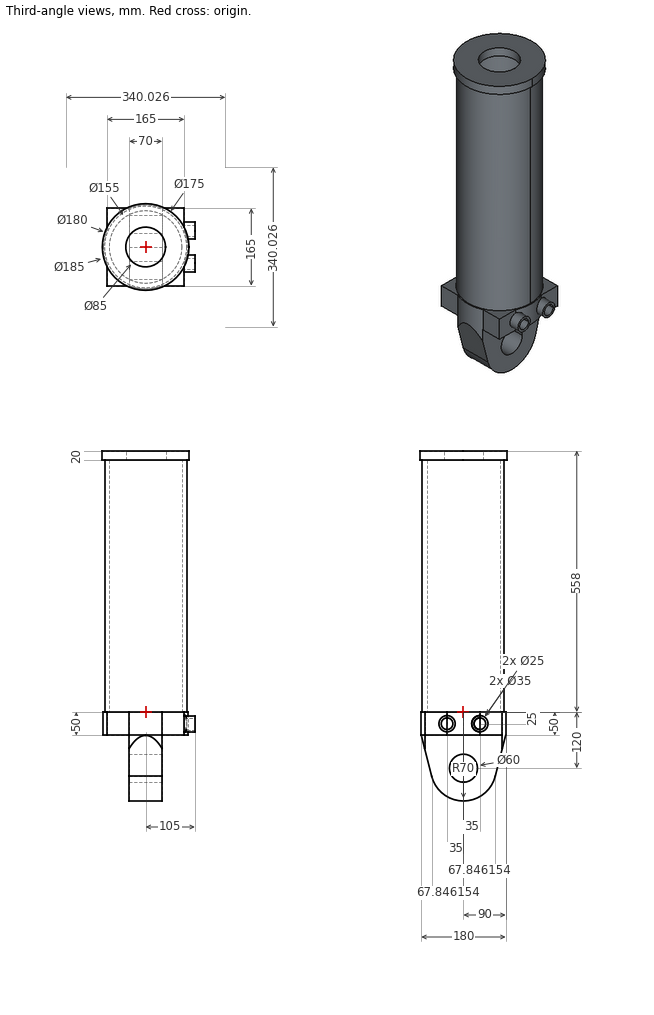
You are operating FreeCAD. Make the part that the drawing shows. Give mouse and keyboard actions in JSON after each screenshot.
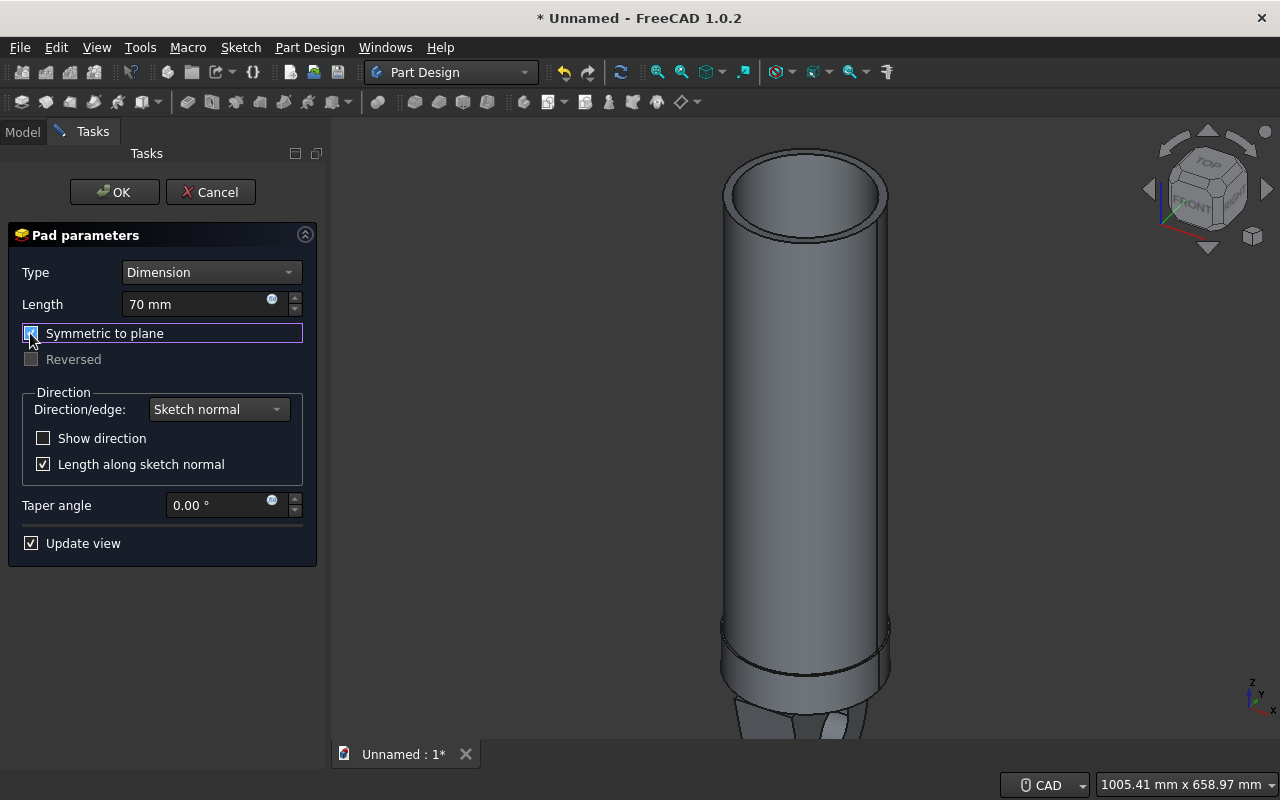
{"action": "left_click", "coordinate": [115, 192]}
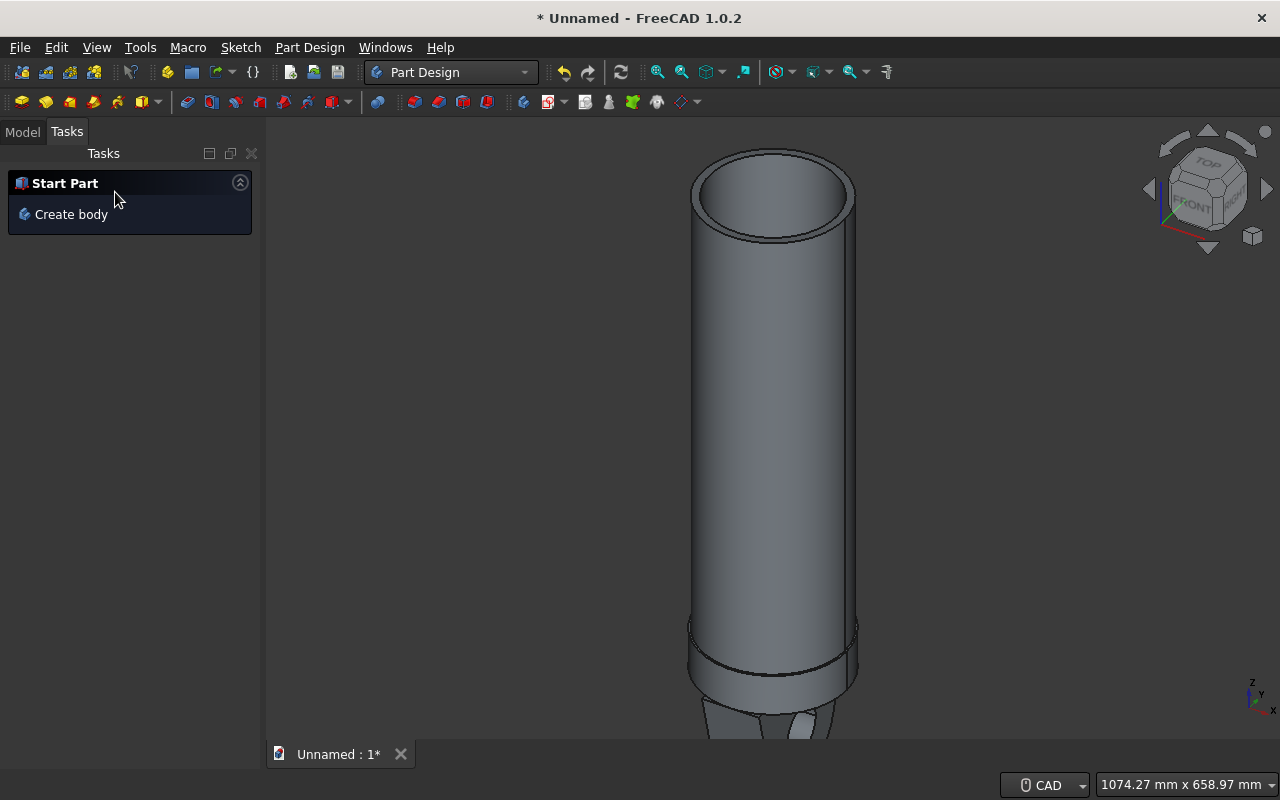
{"action": "key", "text": "v f"}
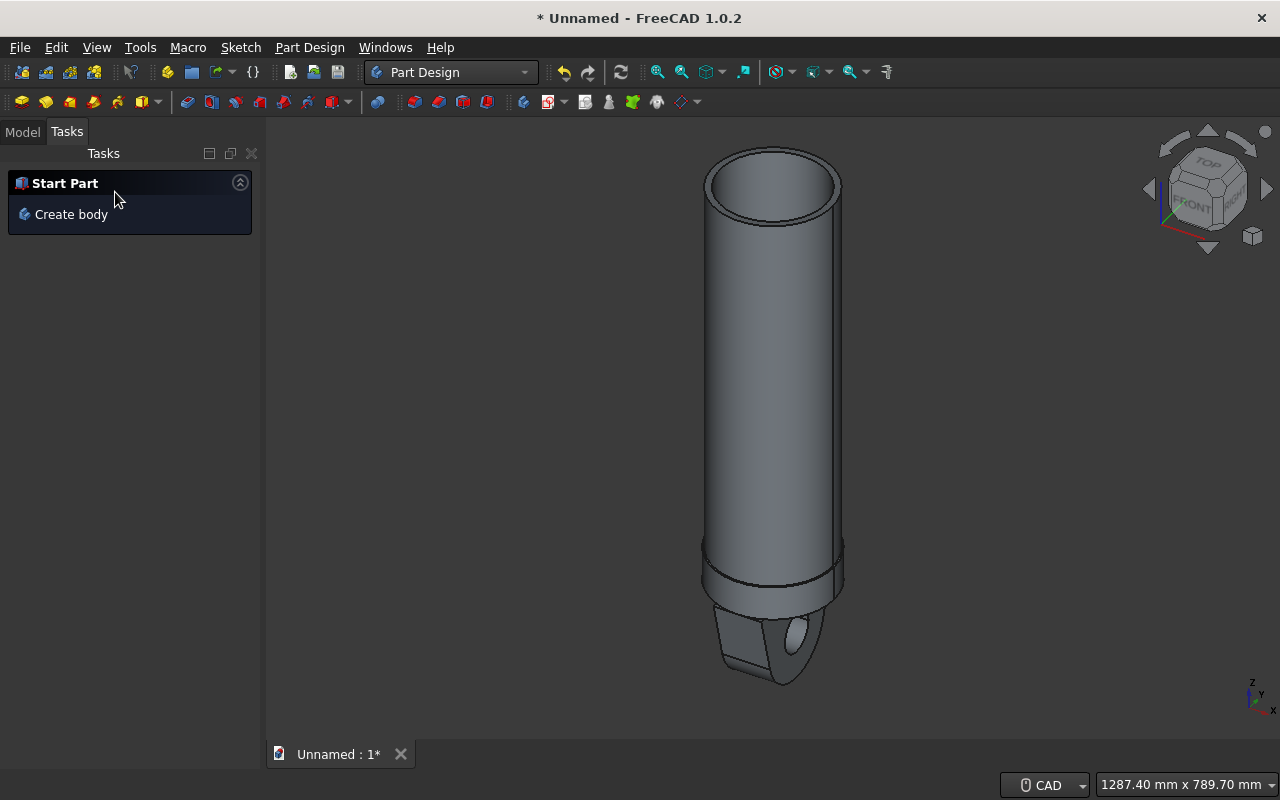
{"action": "key", "text": "5"}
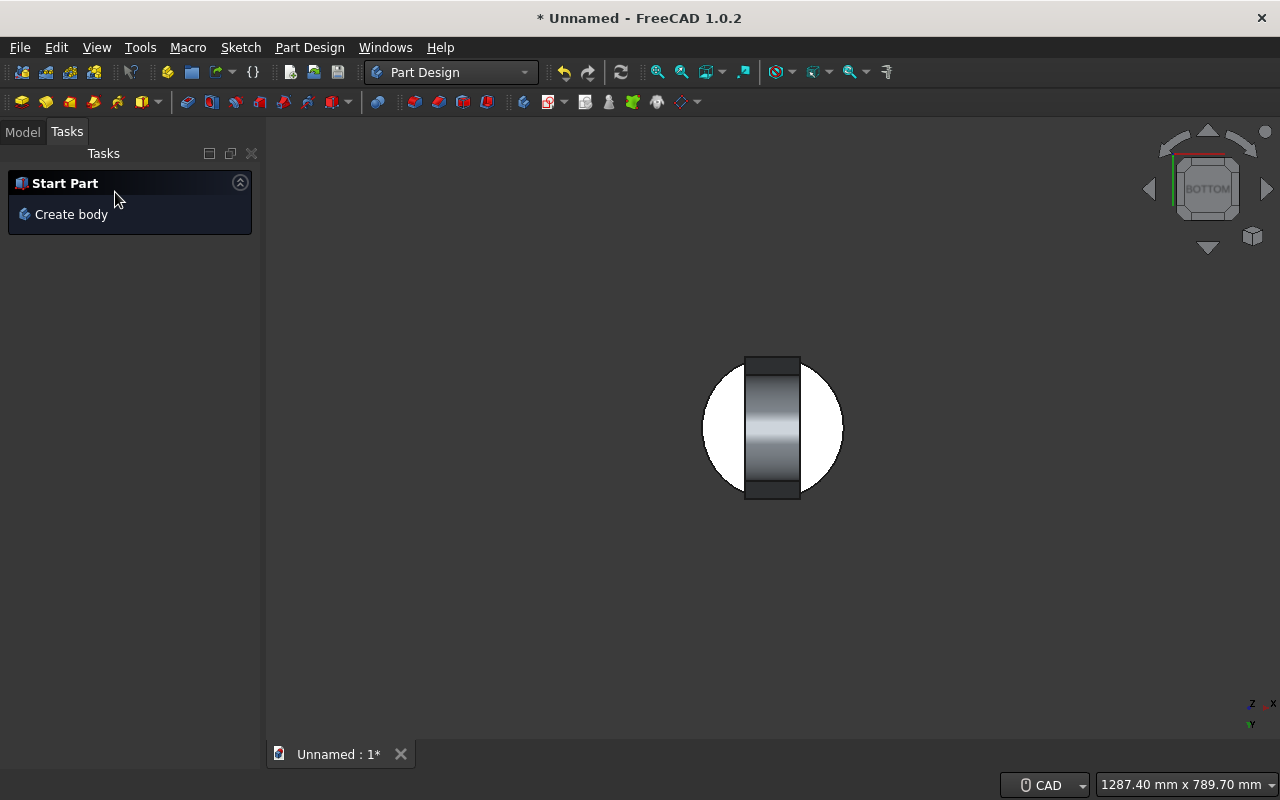
{"action": "left_click", "coordinate": [658, 72]}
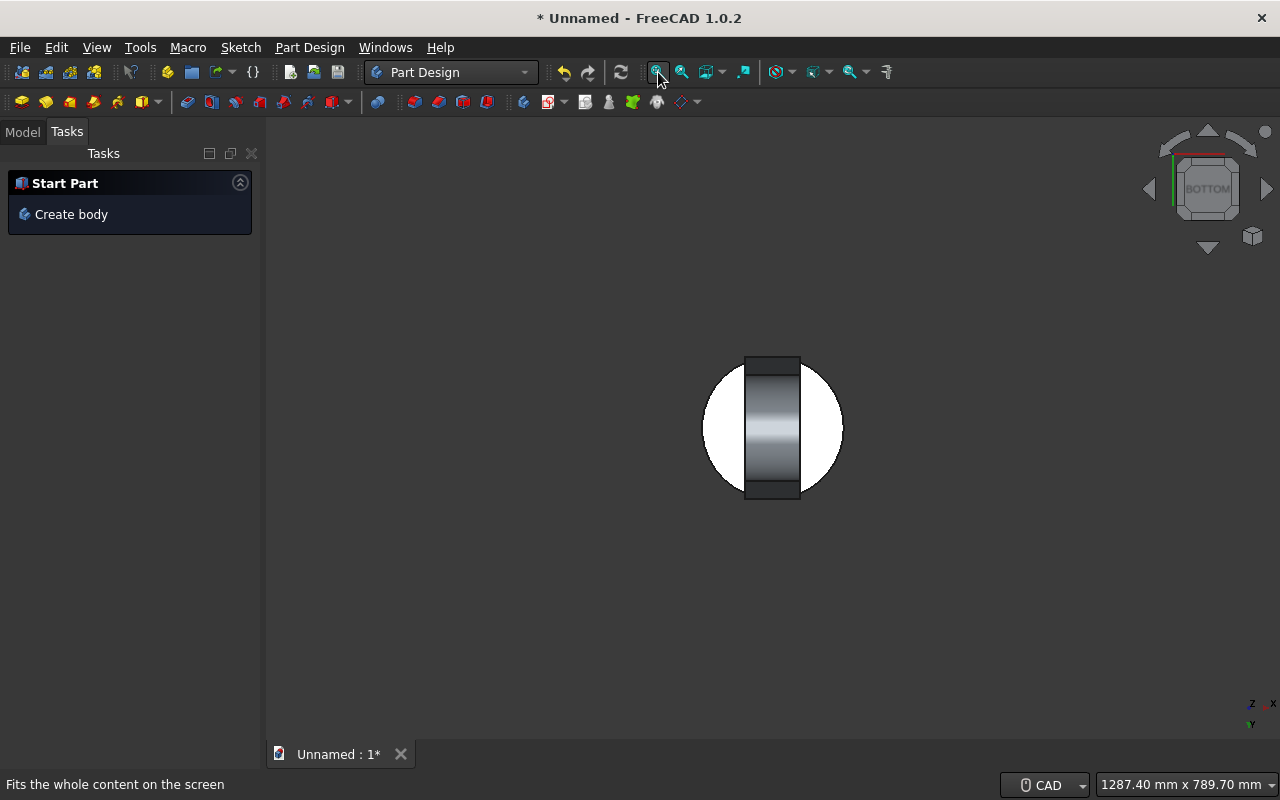
{"action": "left_click", "coordinate": [822, 427]}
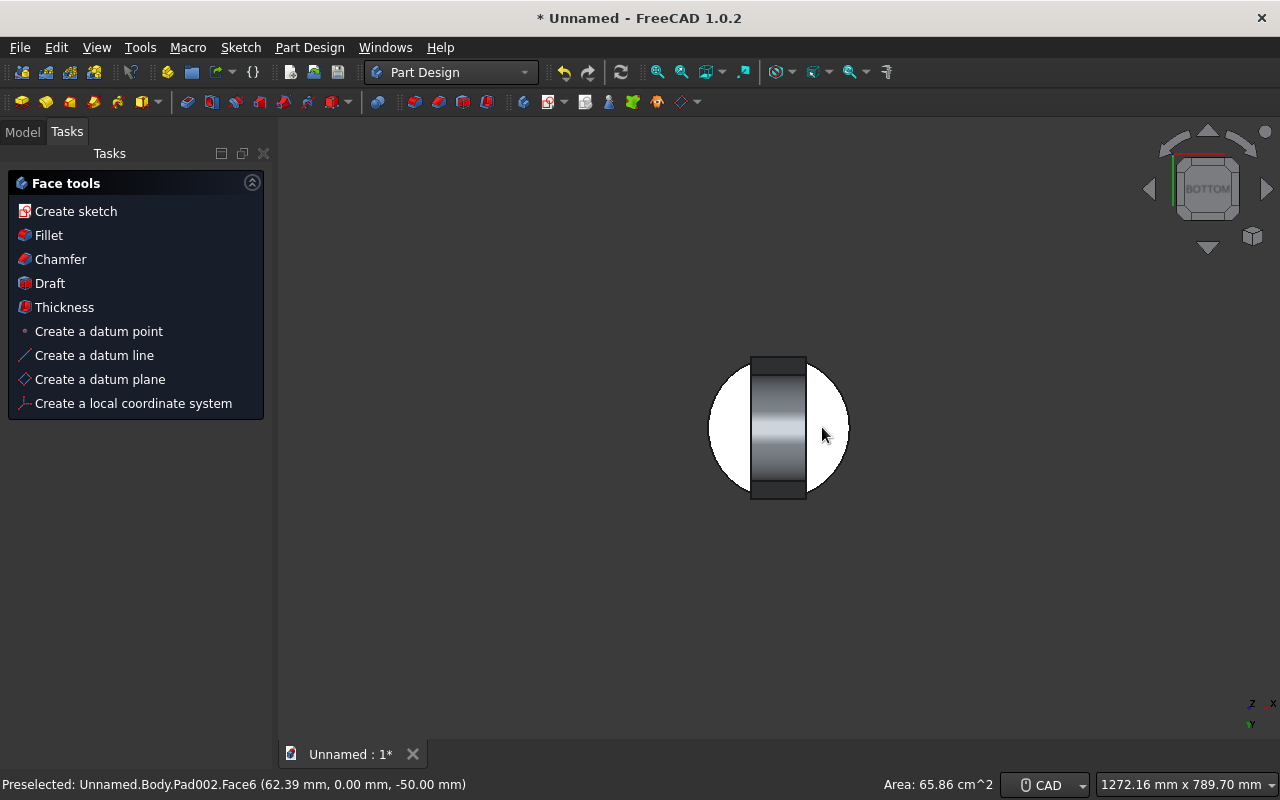
{"action": "left_click", "coordinate": [548, 102]}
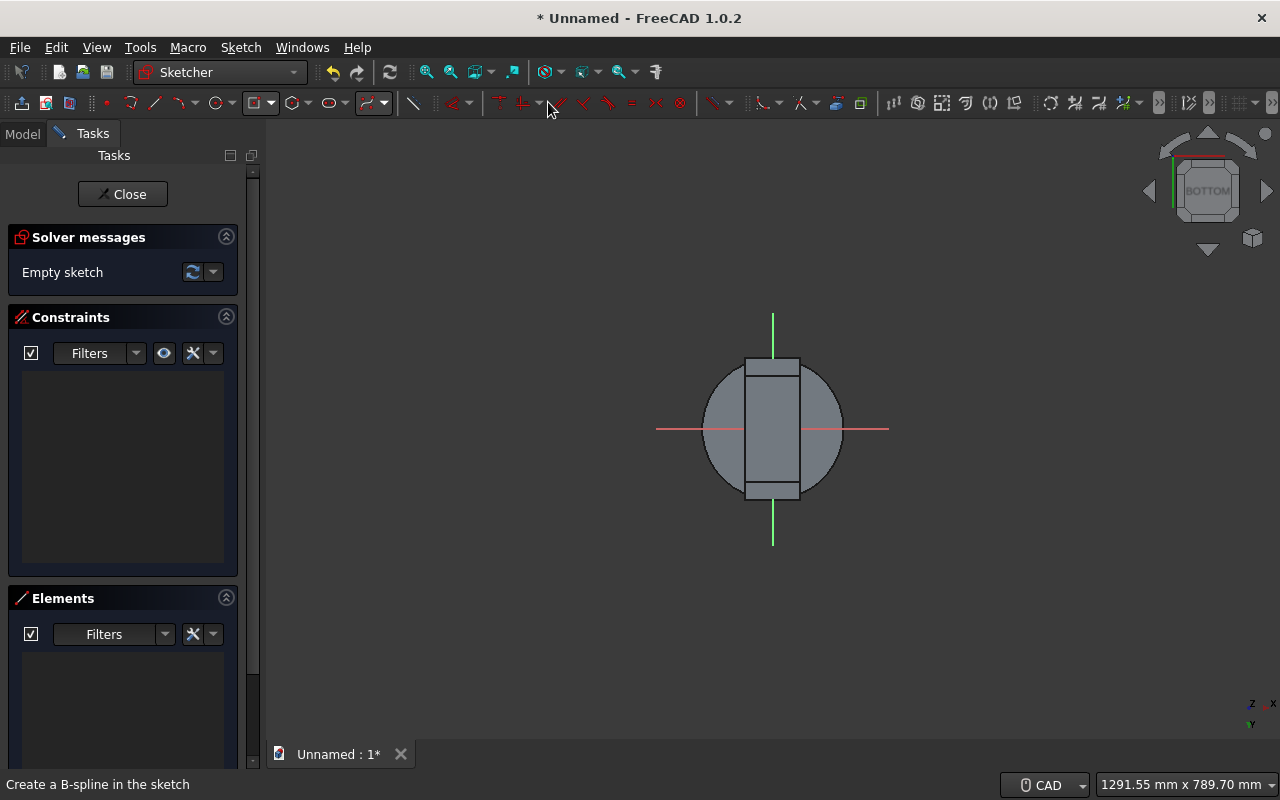
{"action": "left_click", "coordinate": [70, 104]}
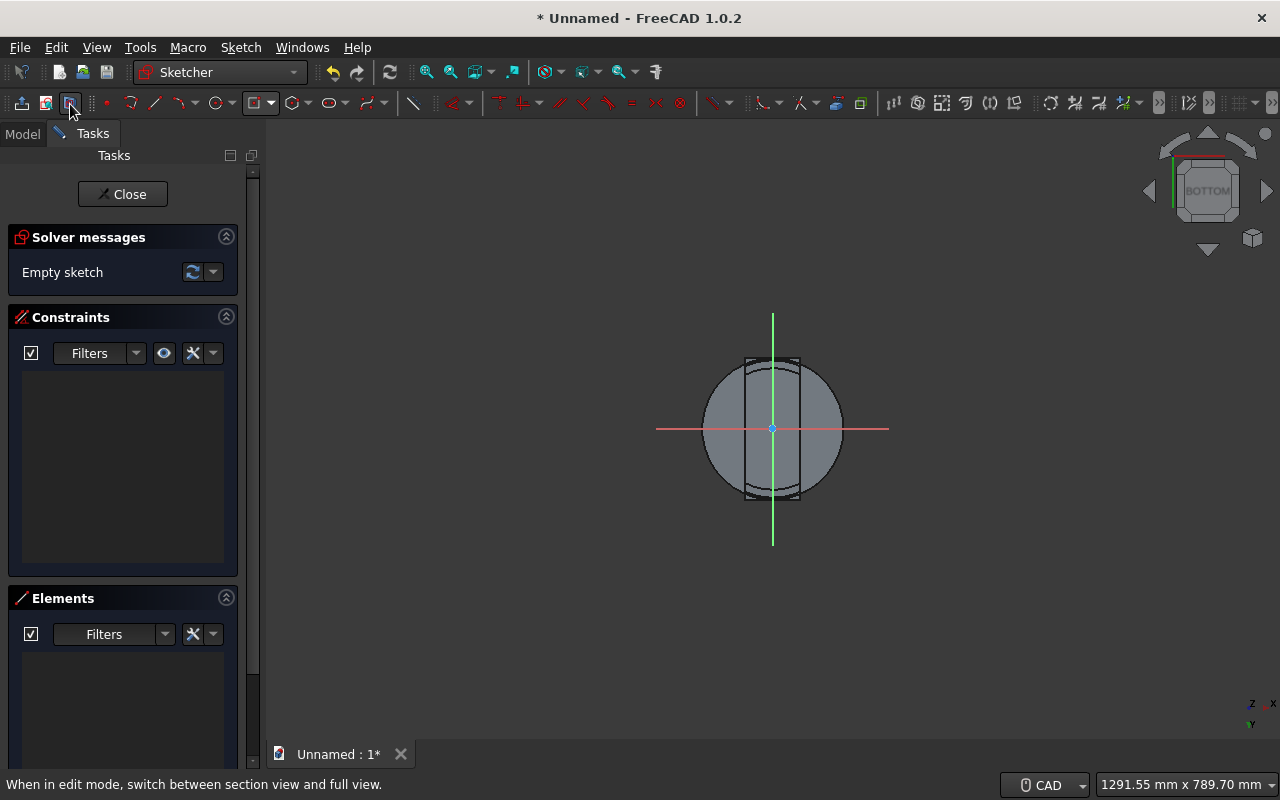
{"action": "scroll", "coordinate": [912, 429], "scroll_direction": "up", "scroll_amount": 2}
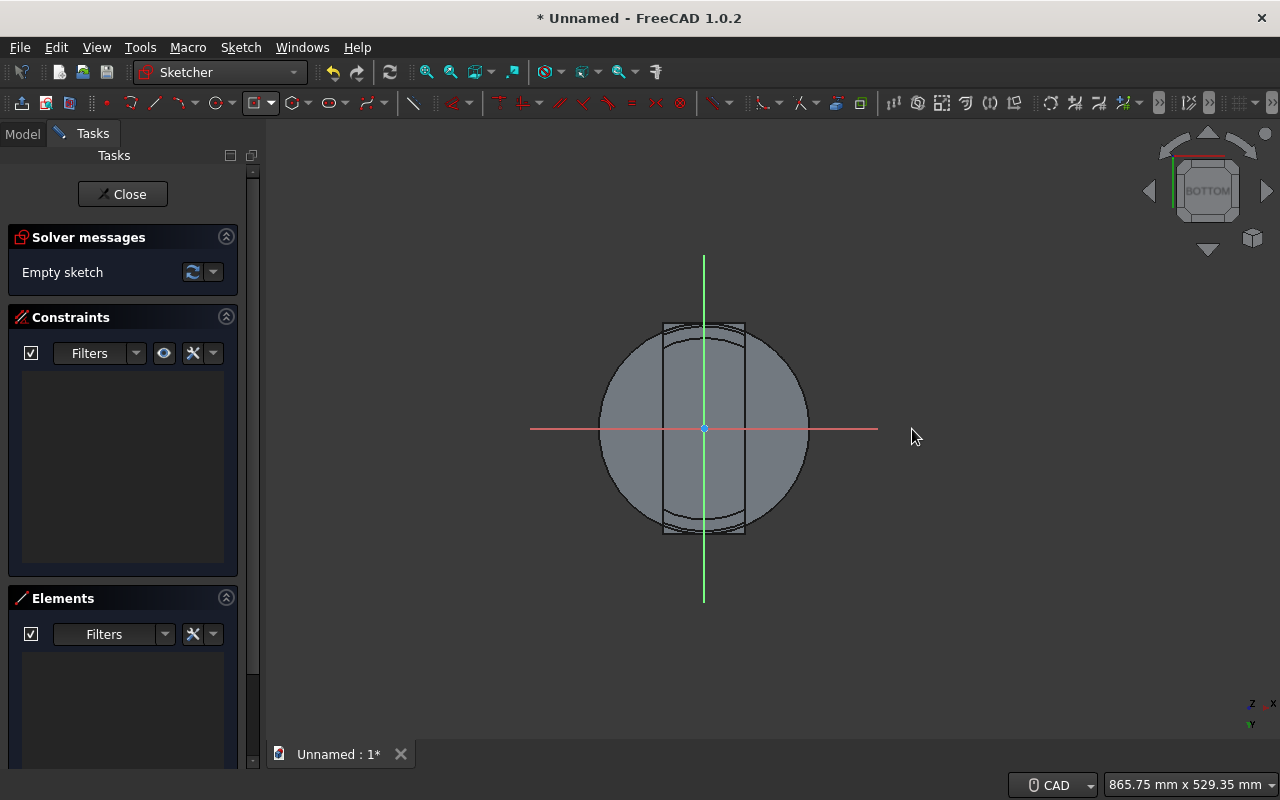
{"action": "key", "text": "g v"}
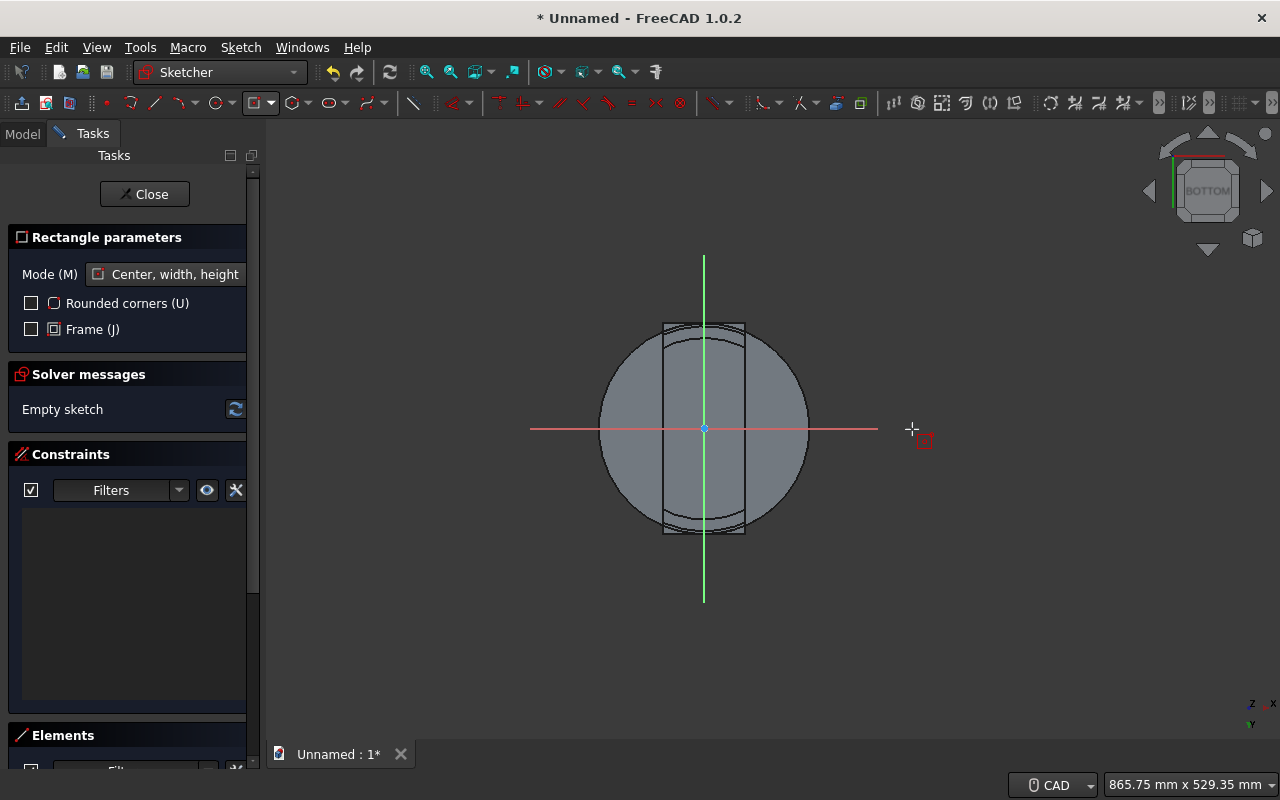
{"action": "left_click", "coordinate": [704, 429]}
{"action": "left_click", "coordinate": [903, 230]}